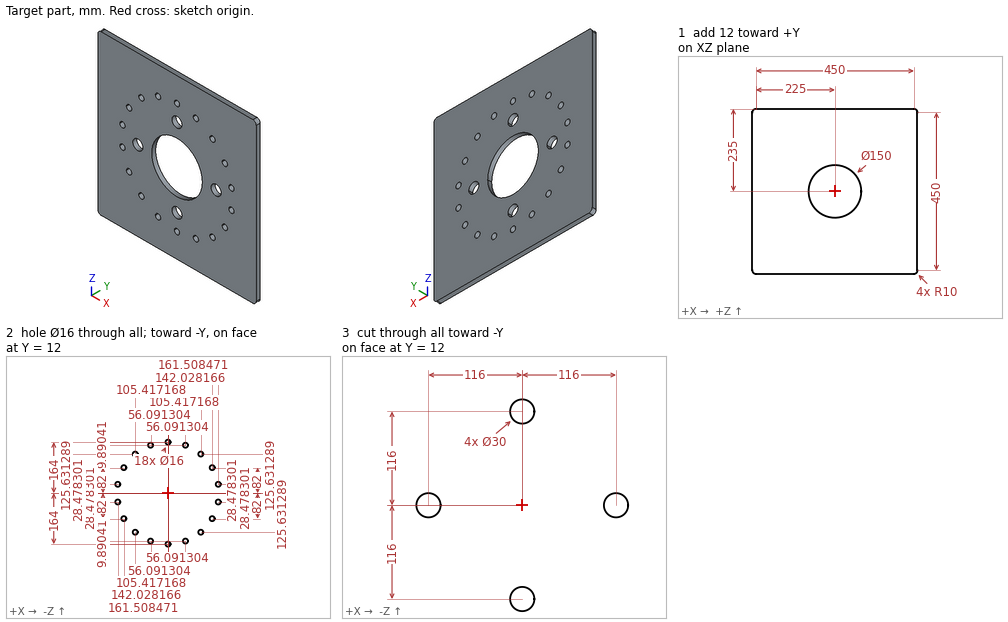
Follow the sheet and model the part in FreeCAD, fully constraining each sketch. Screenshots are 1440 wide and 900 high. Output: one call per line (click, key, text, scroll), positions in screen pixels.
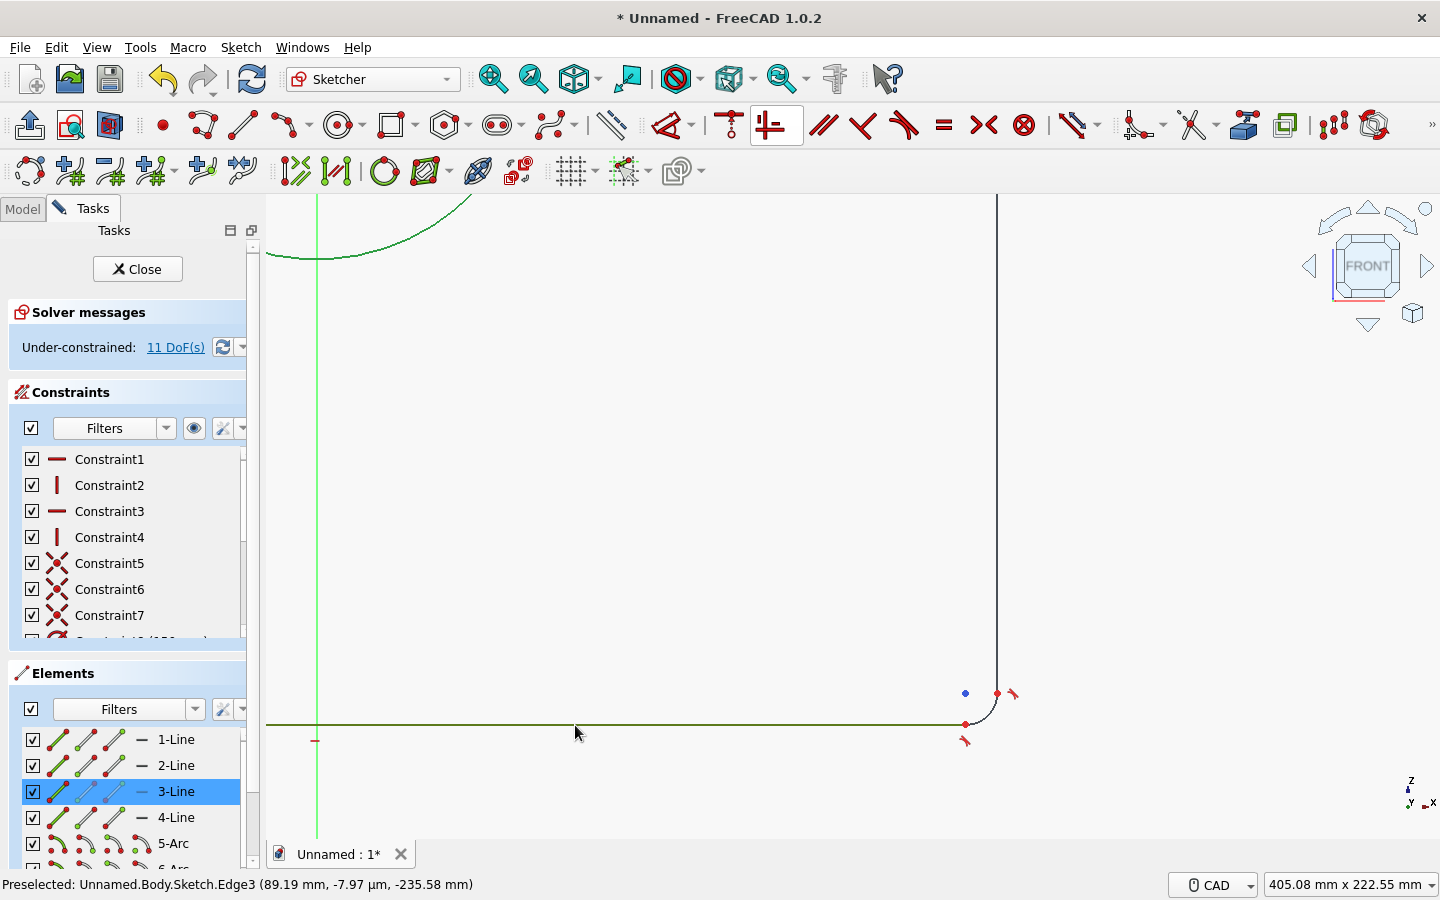
scroll(986, 721, down, 6)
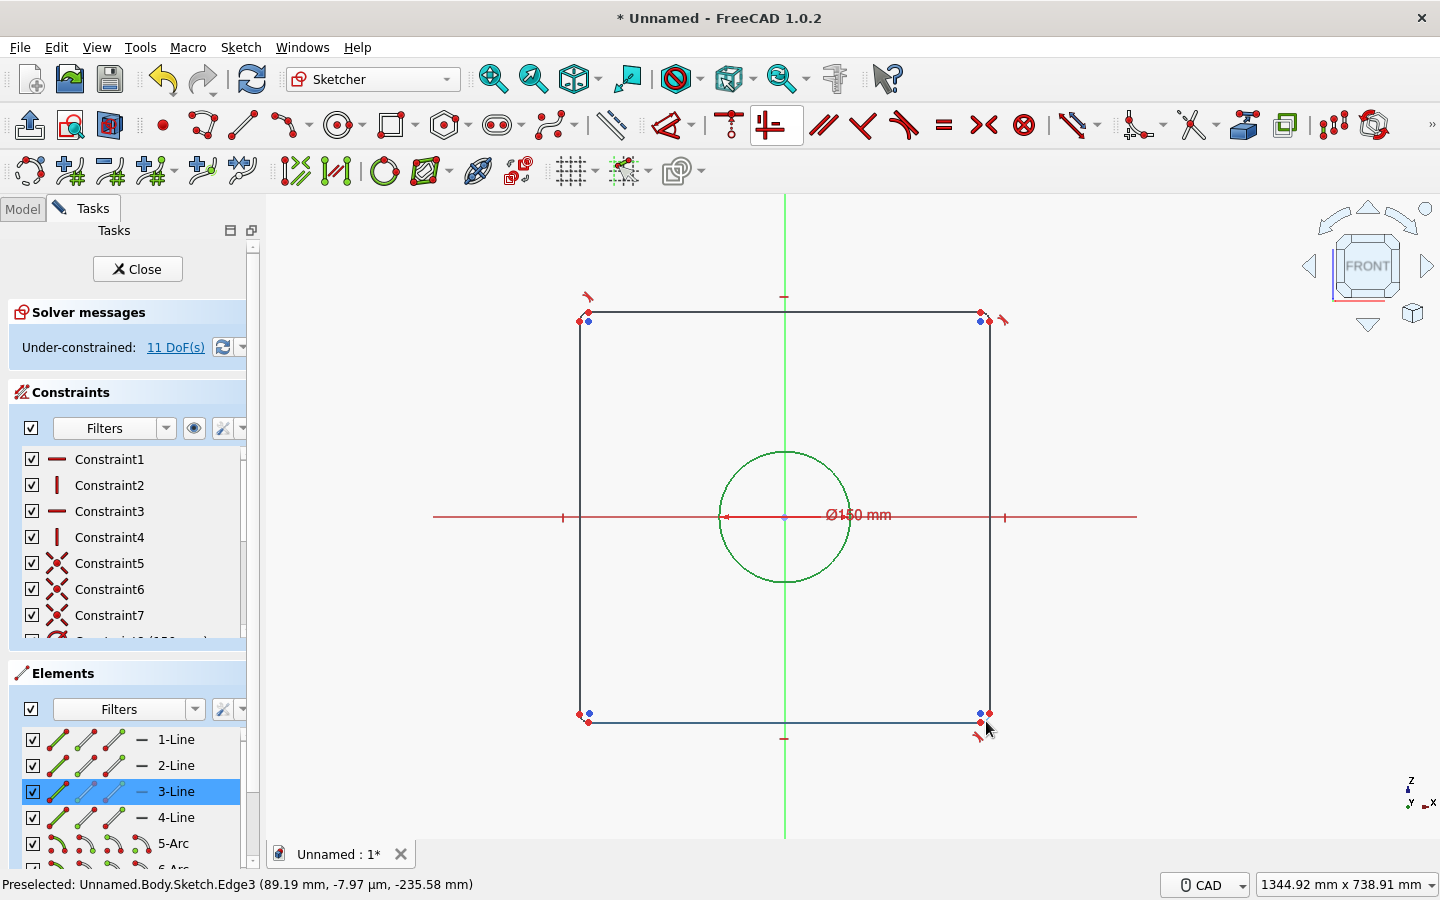
scroll(581, 718, up, 7)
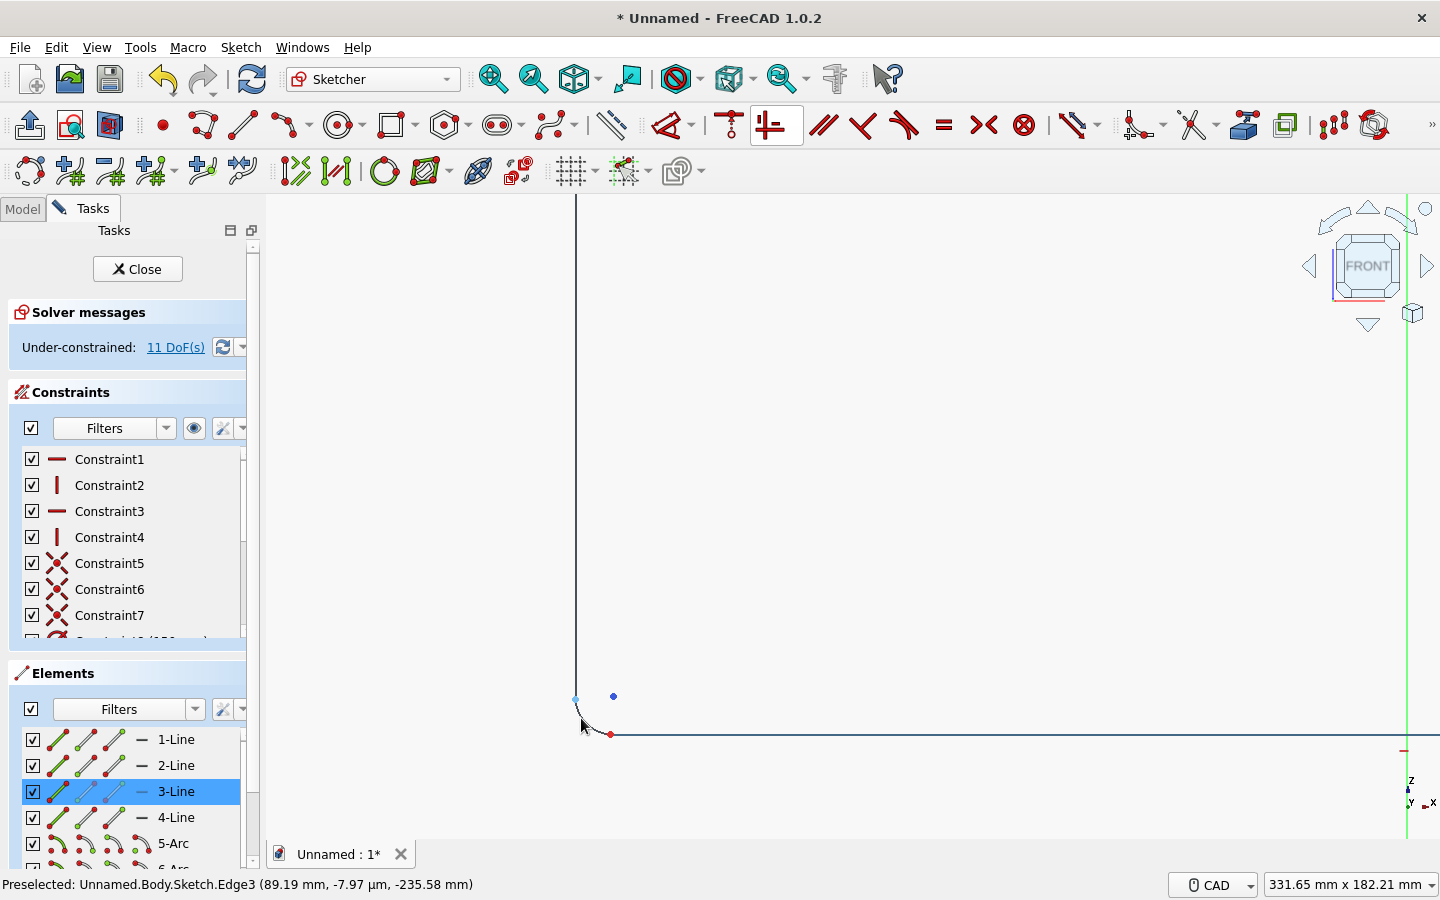
click(580, 715)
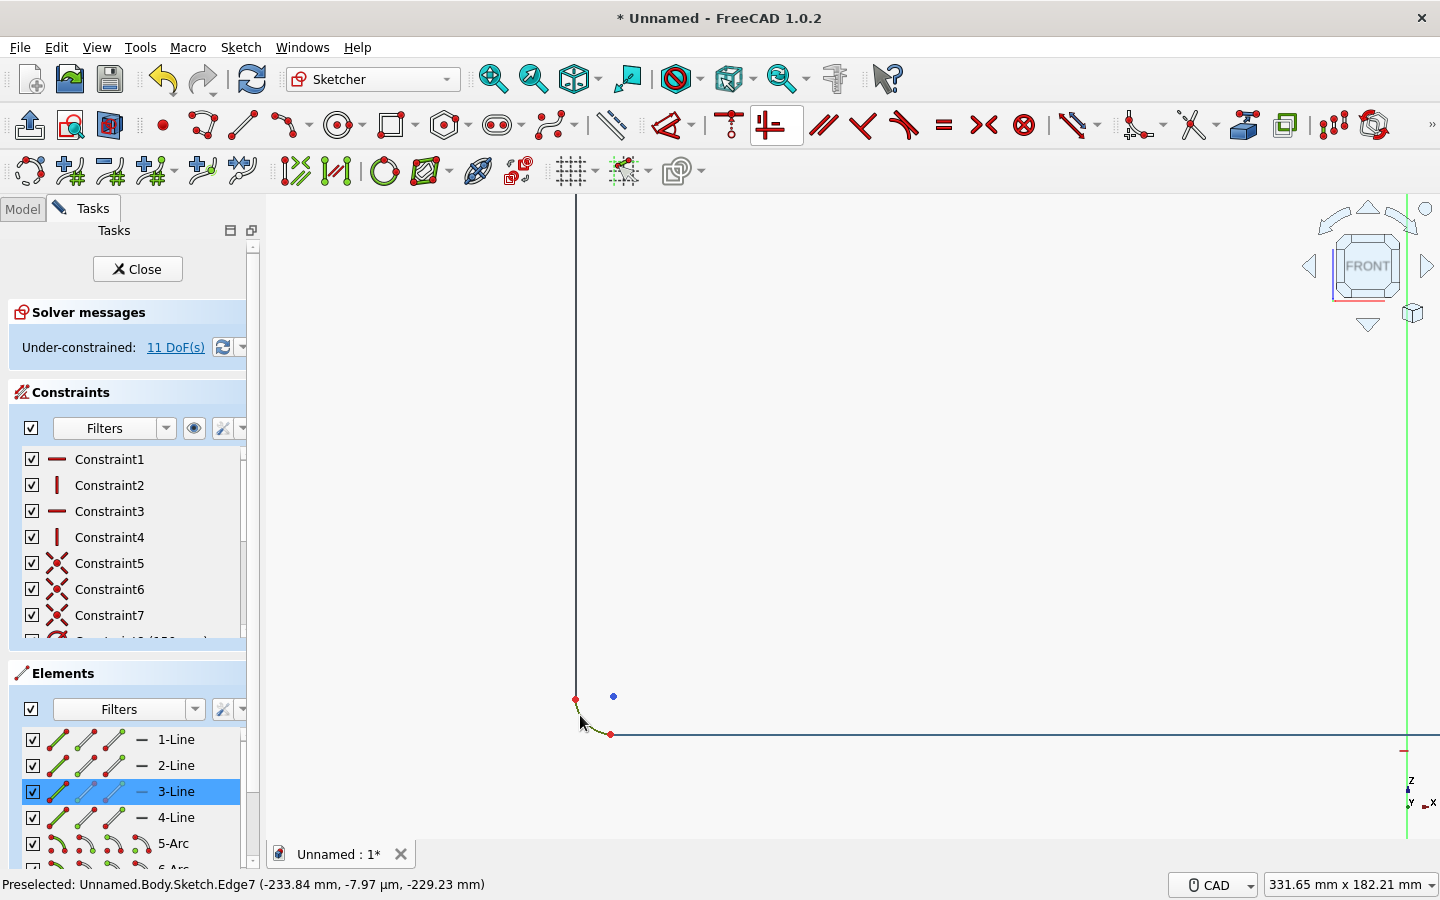
key(t)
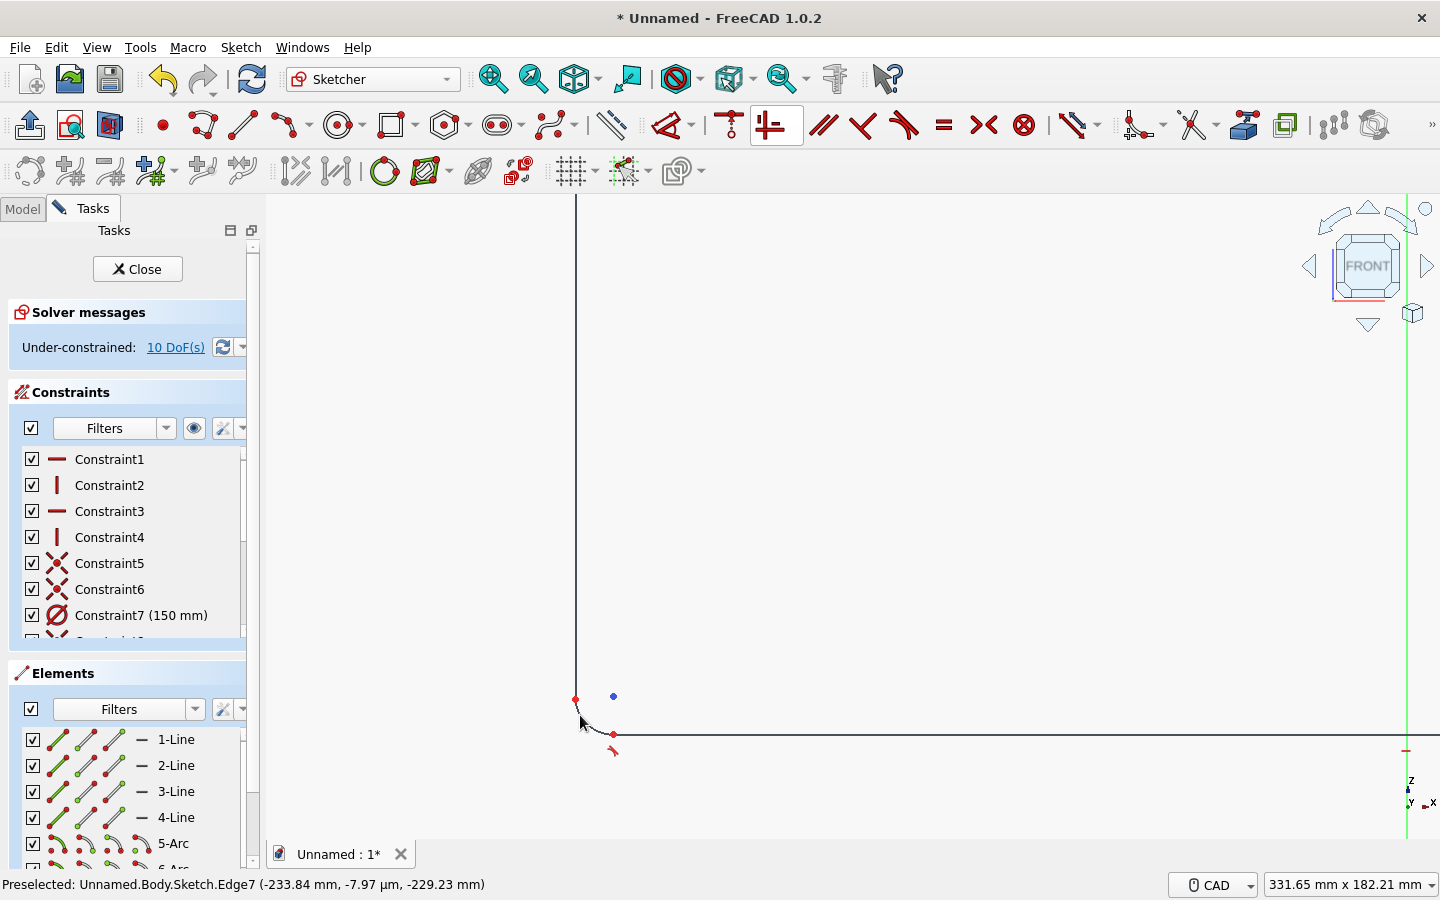
scroll(581, 718, down, 7)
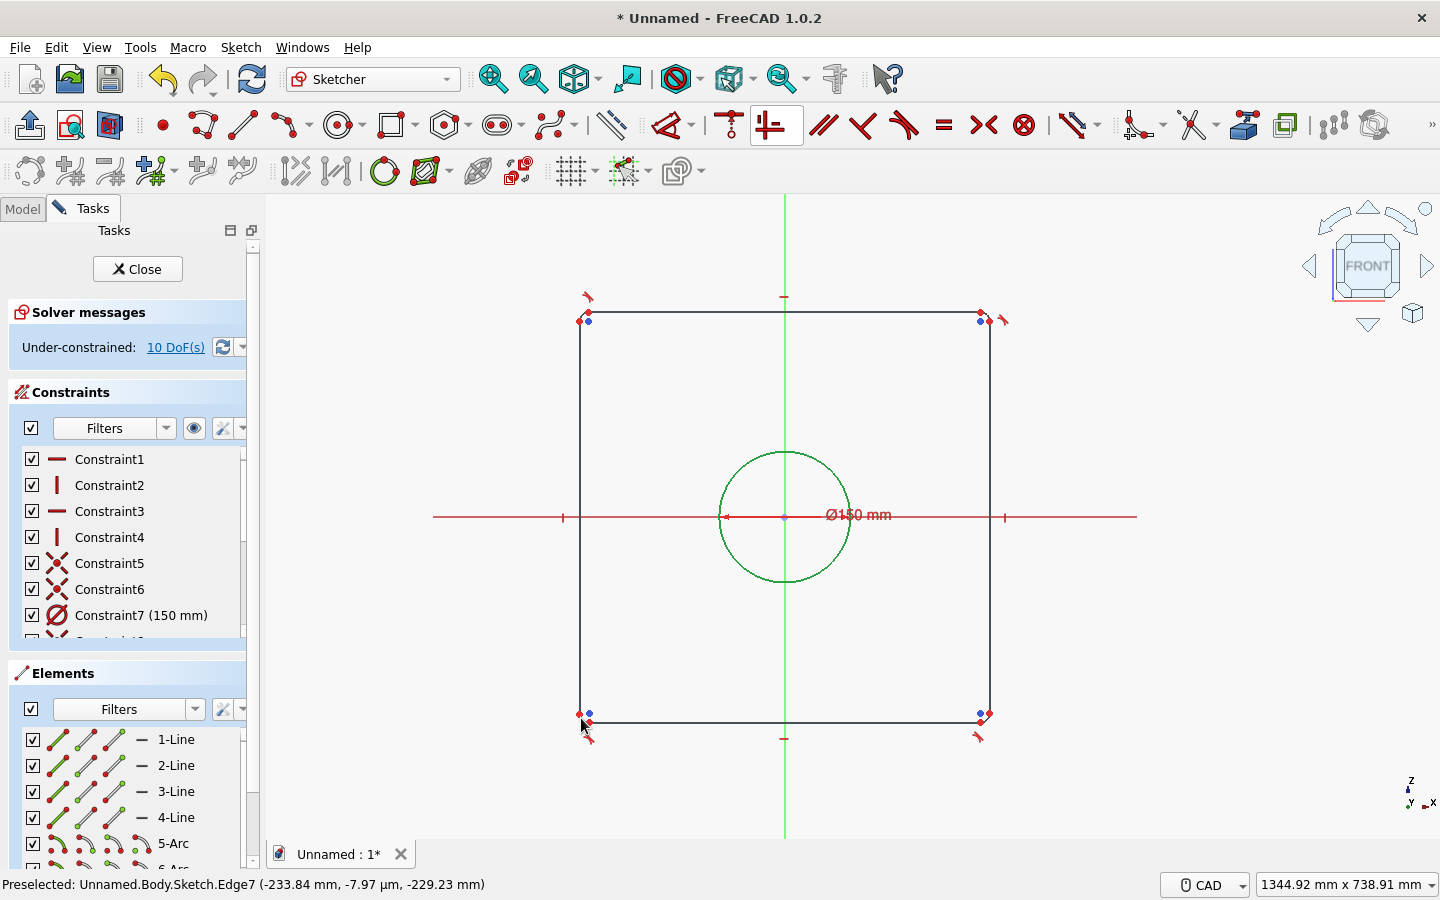
click(580, 596)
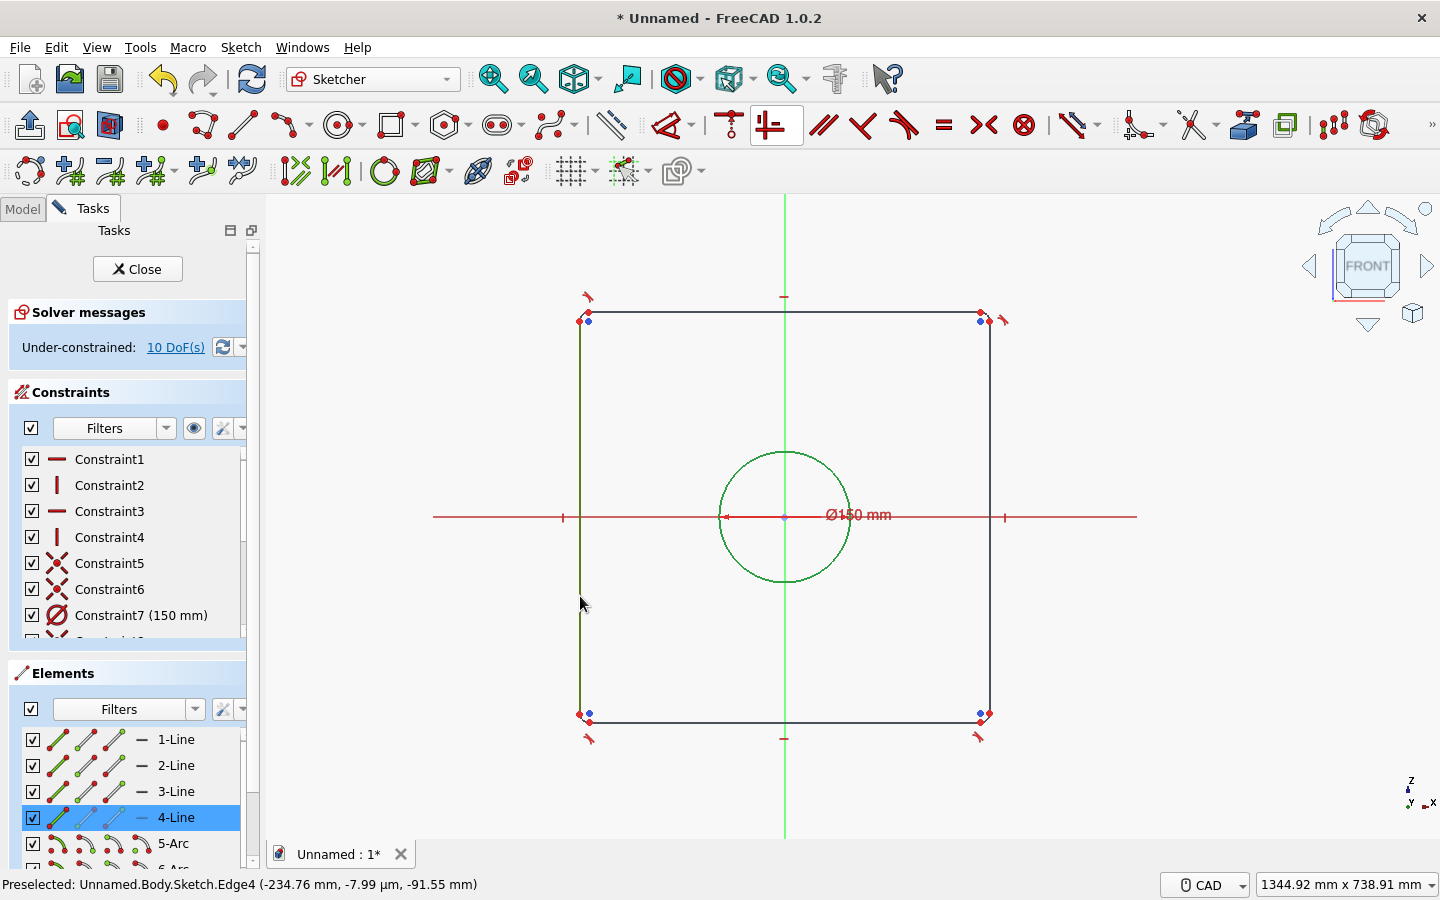
scroll(583, 720, up, 4)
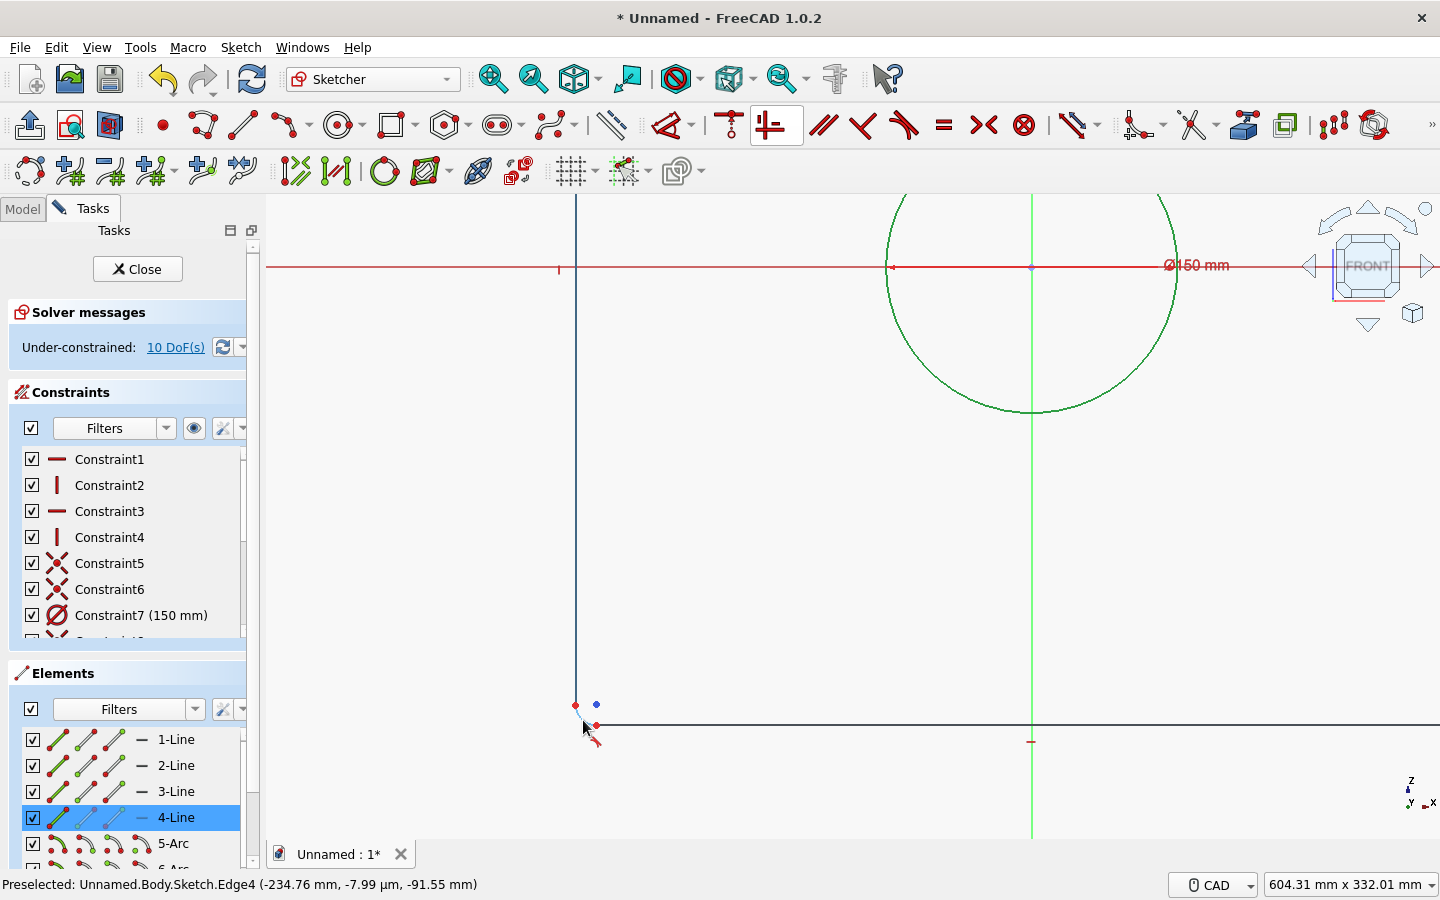
click(582, 720)